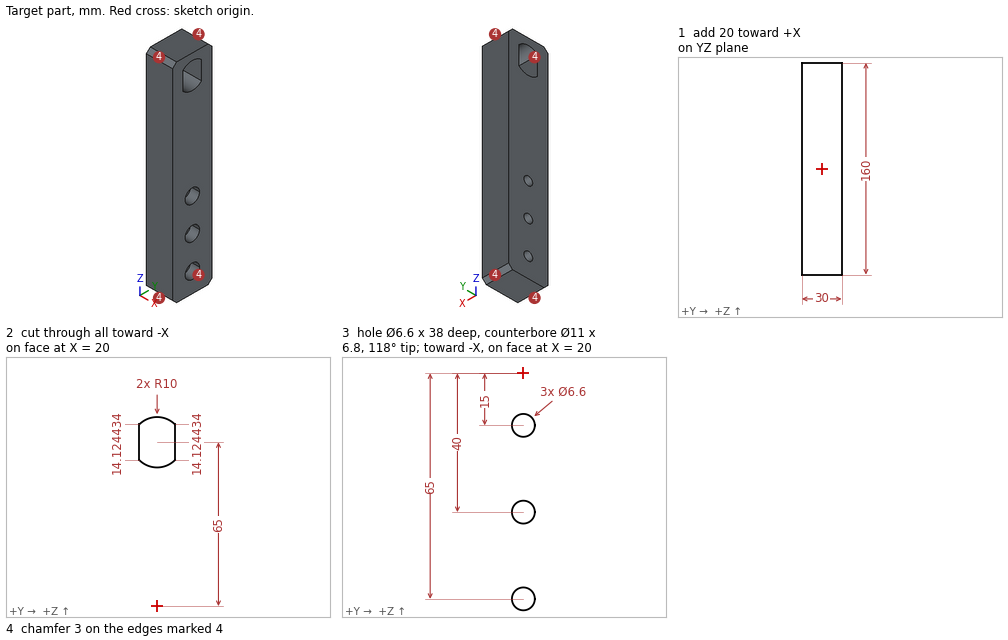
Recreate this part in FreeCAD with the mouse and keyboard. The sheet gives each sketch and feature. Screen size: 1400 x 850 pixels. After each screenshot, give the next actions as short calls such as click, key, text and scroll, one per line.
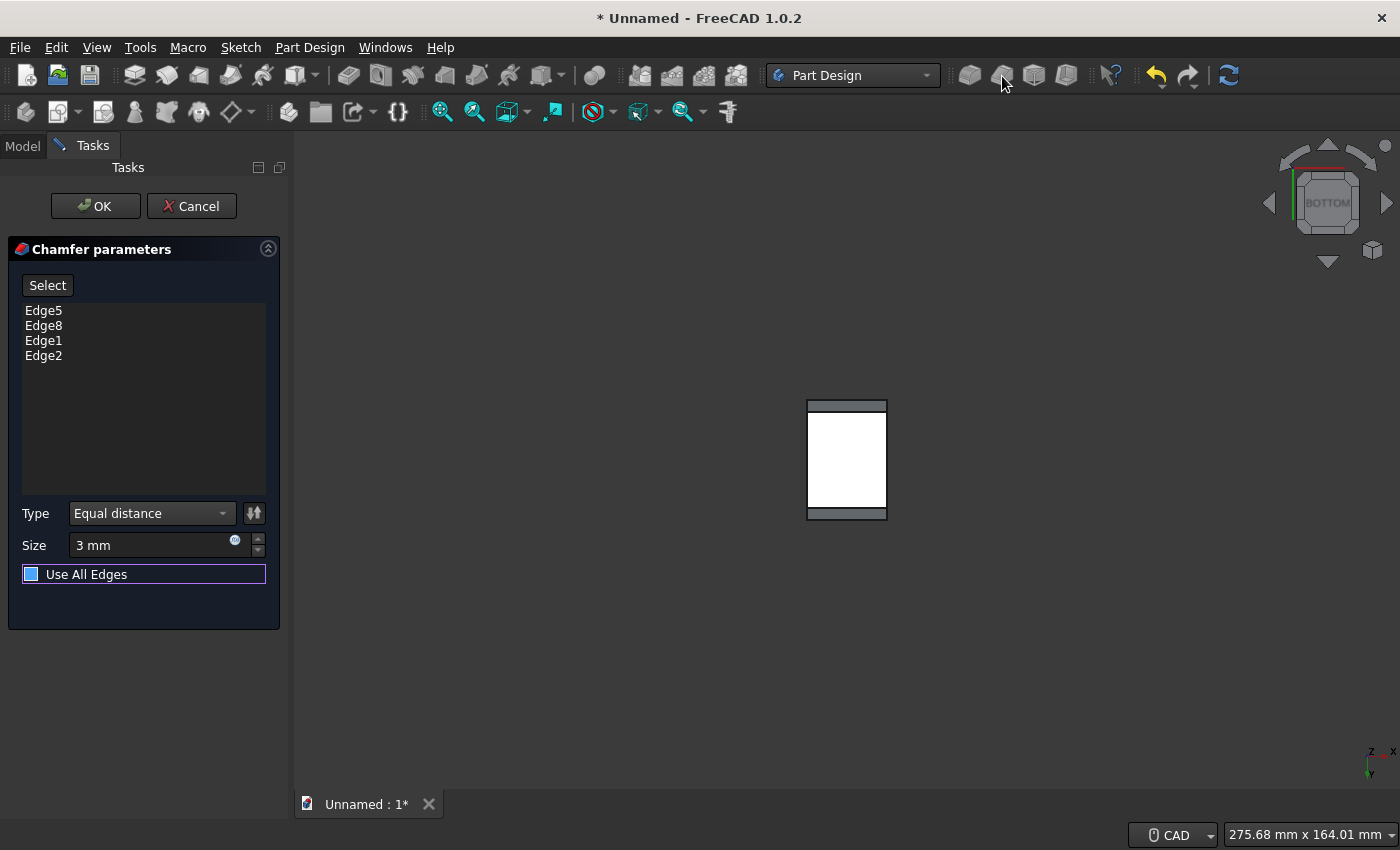
click(96, 206)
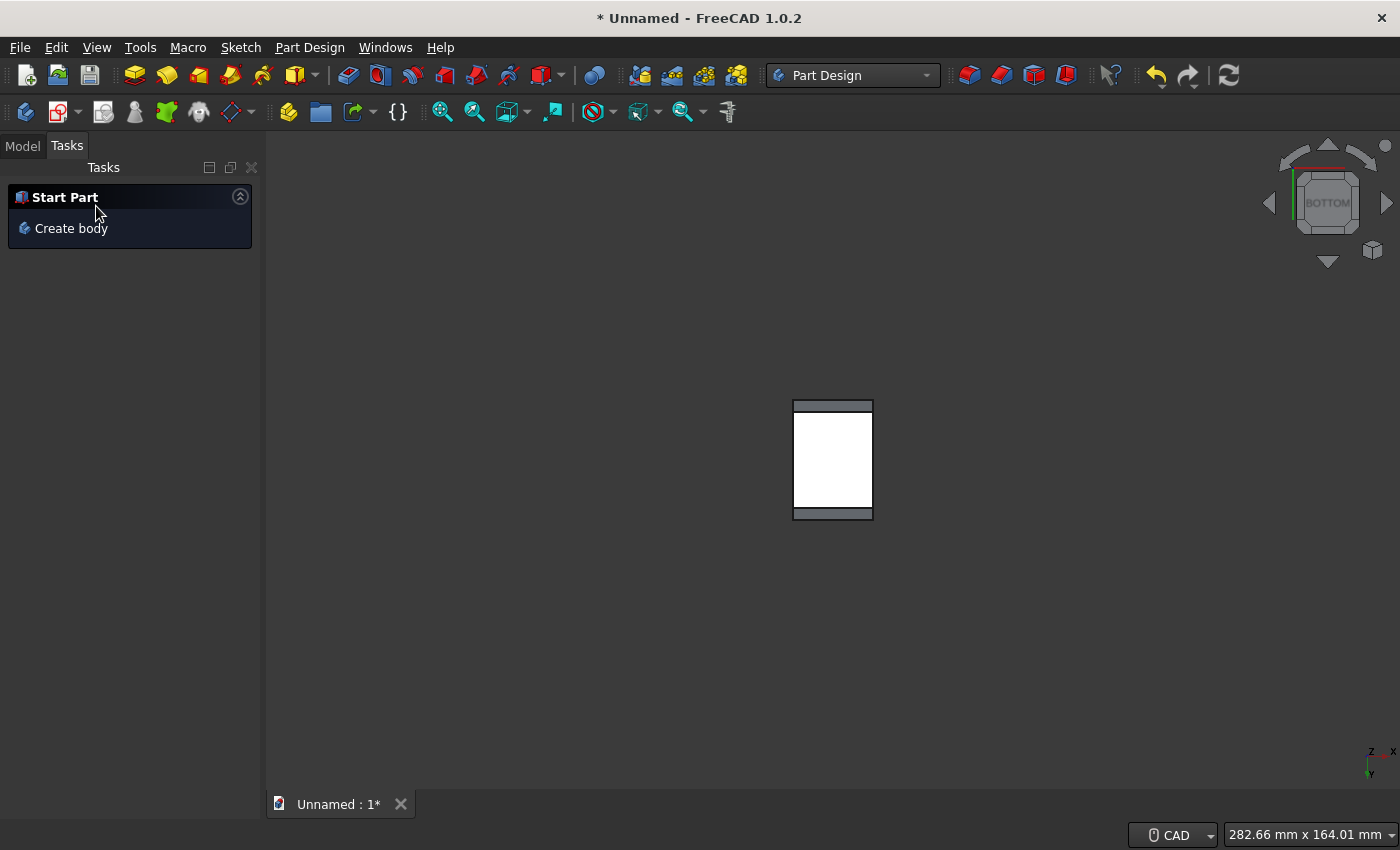
key(0)